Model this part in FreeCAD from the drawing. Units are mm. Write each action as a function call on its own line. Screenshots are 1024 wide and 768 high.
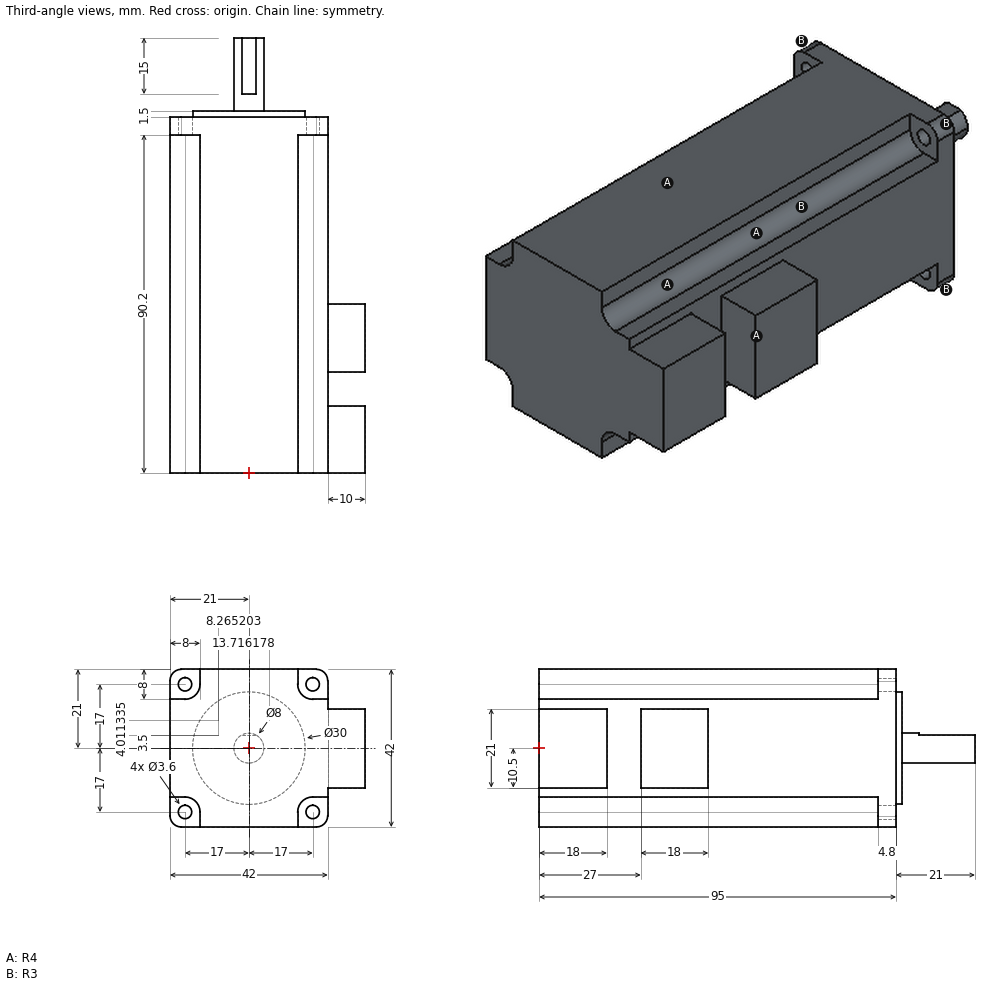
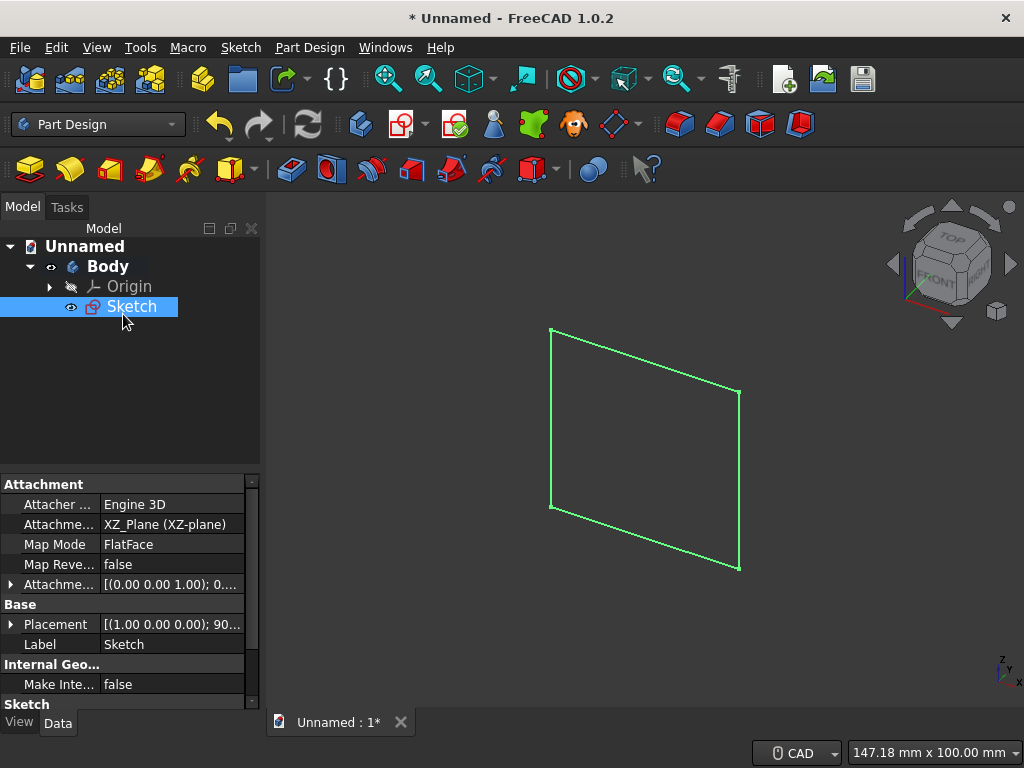
click(30, 170)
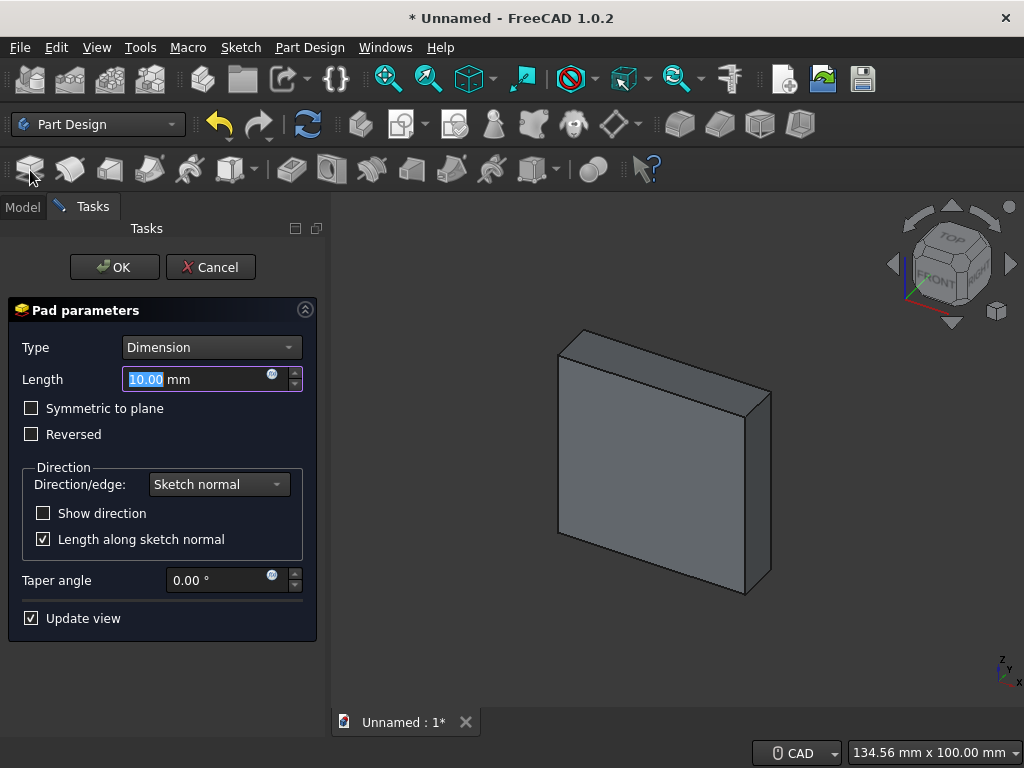
text(95)
key(Tab)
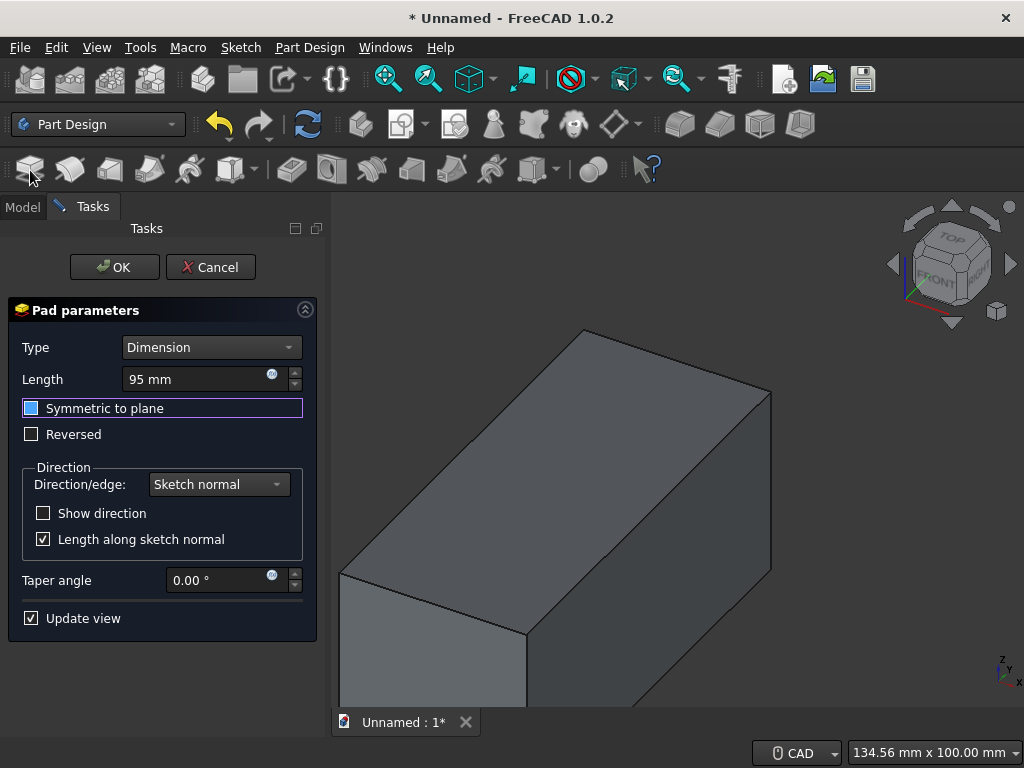
click(30, 434)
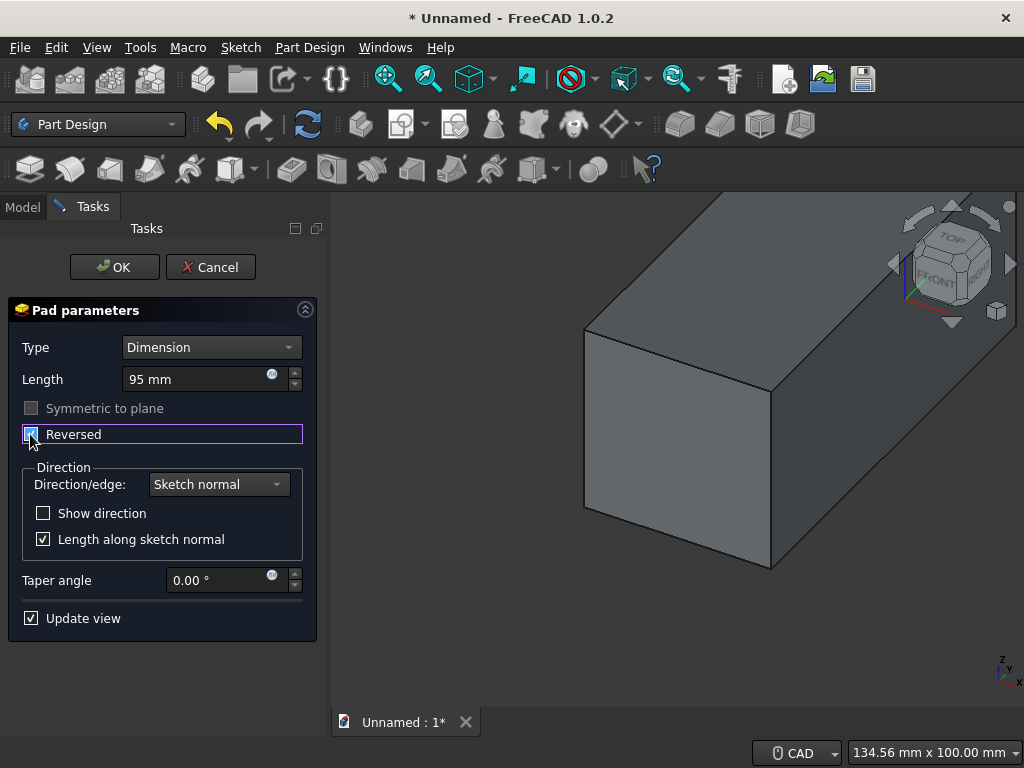
click(115, 267)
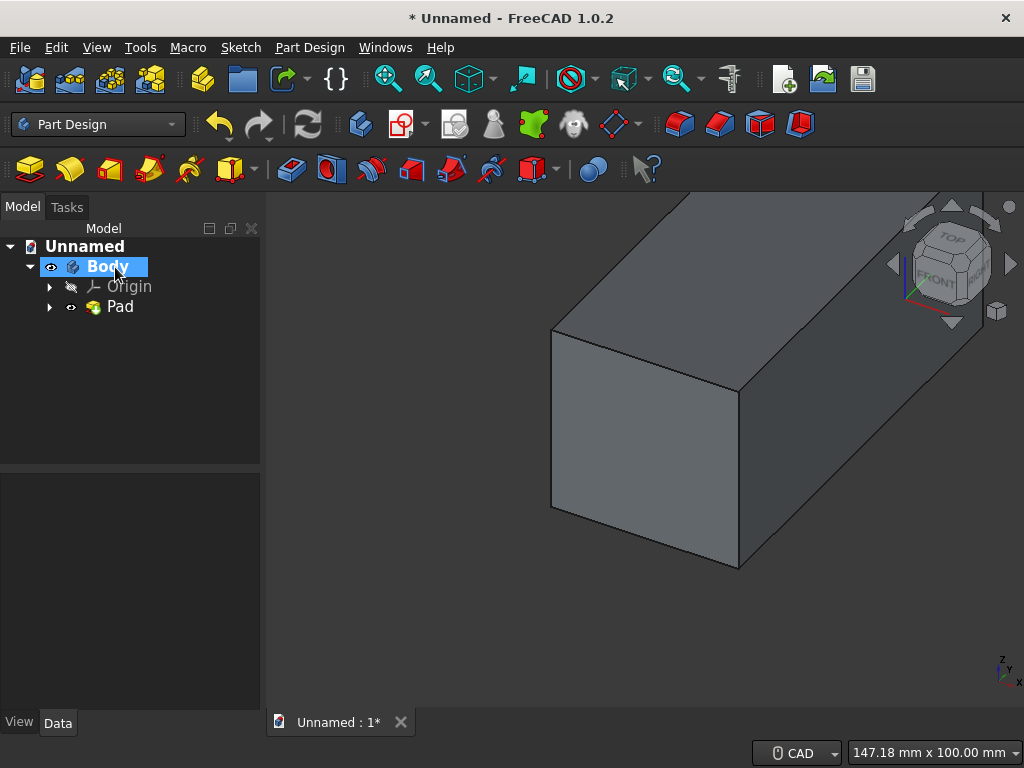
click(390, 80)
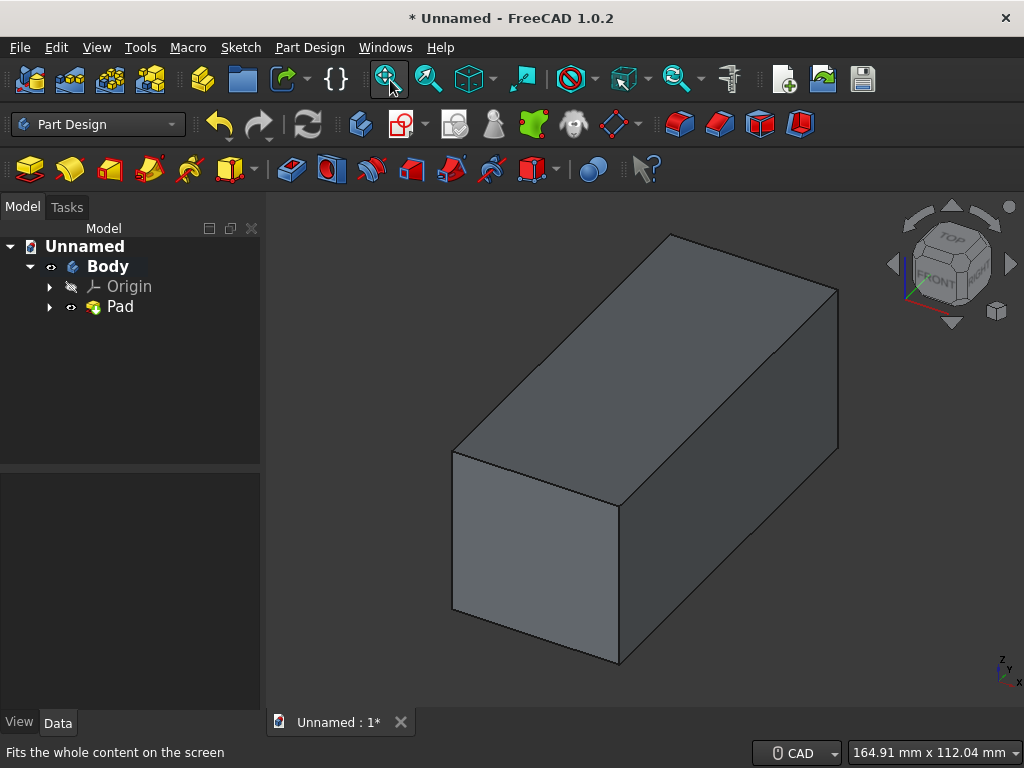
click(536, 557)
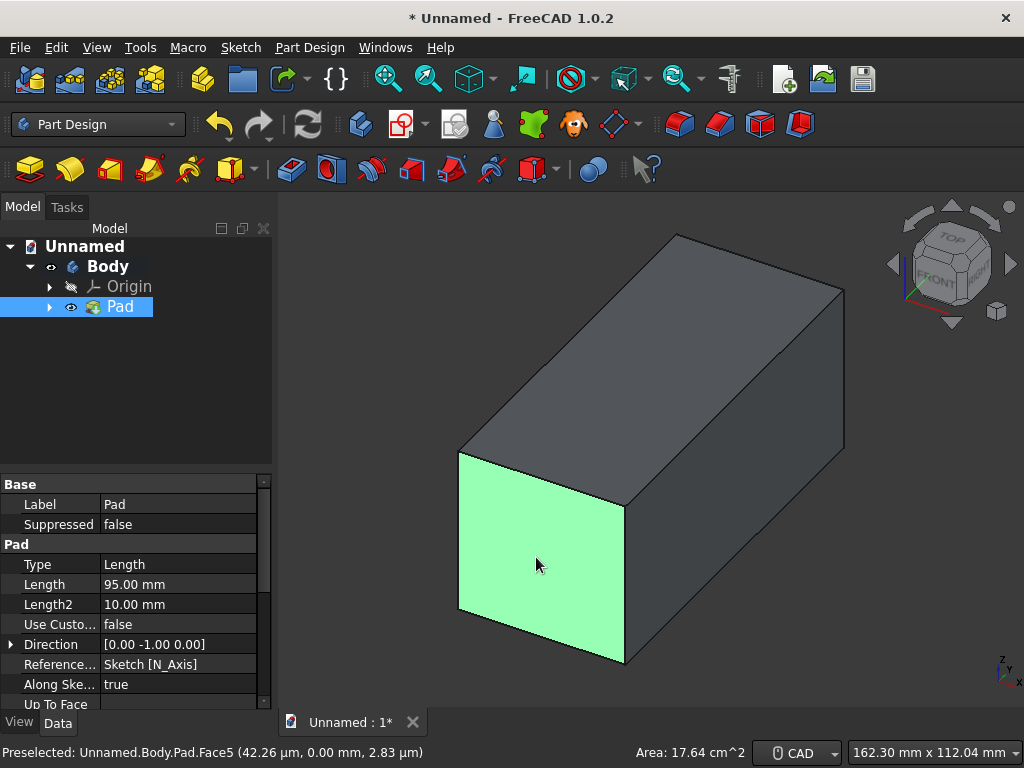
click(402, 124)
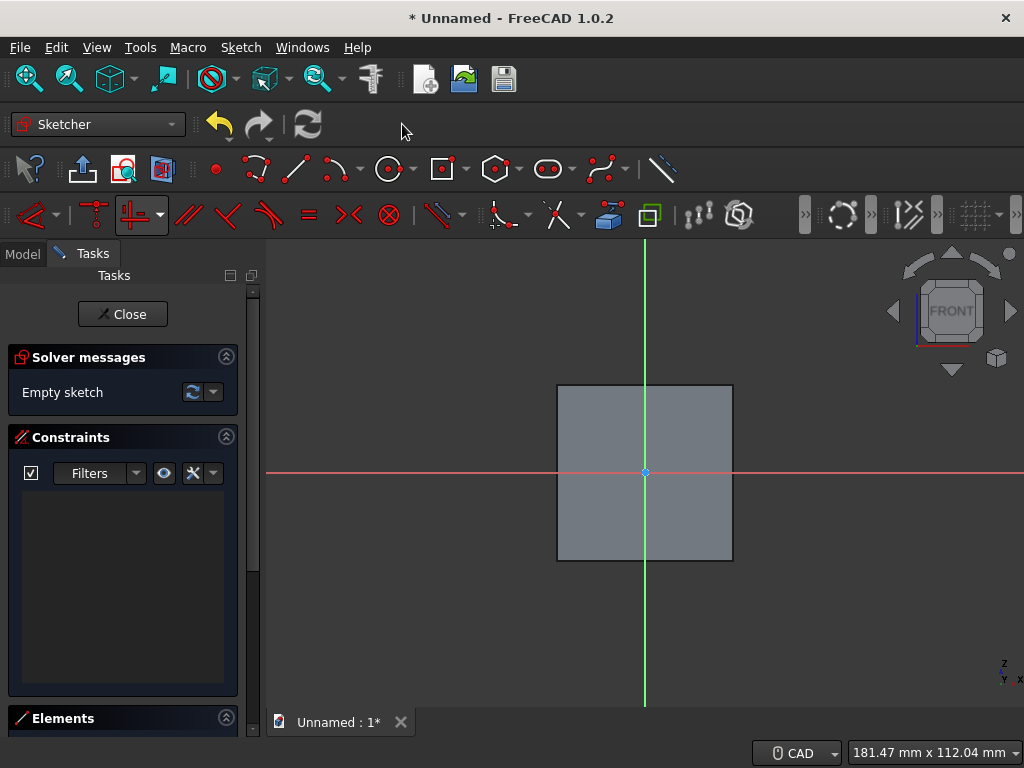
scroll(728, 473, up, 3)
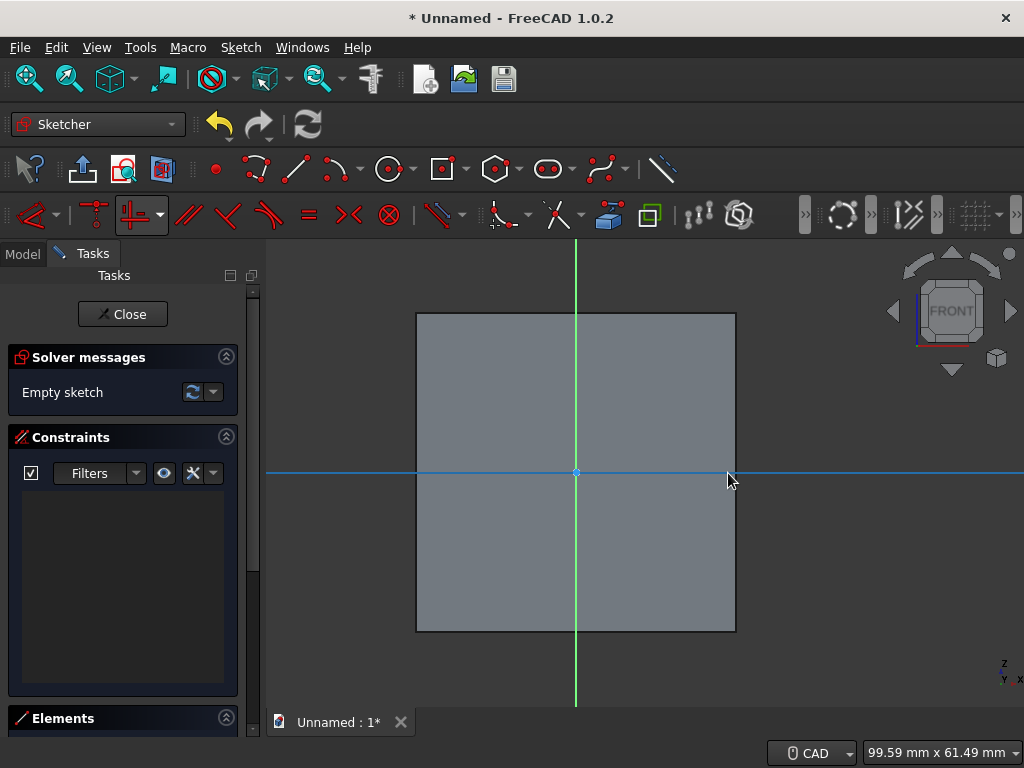
click(468, 170)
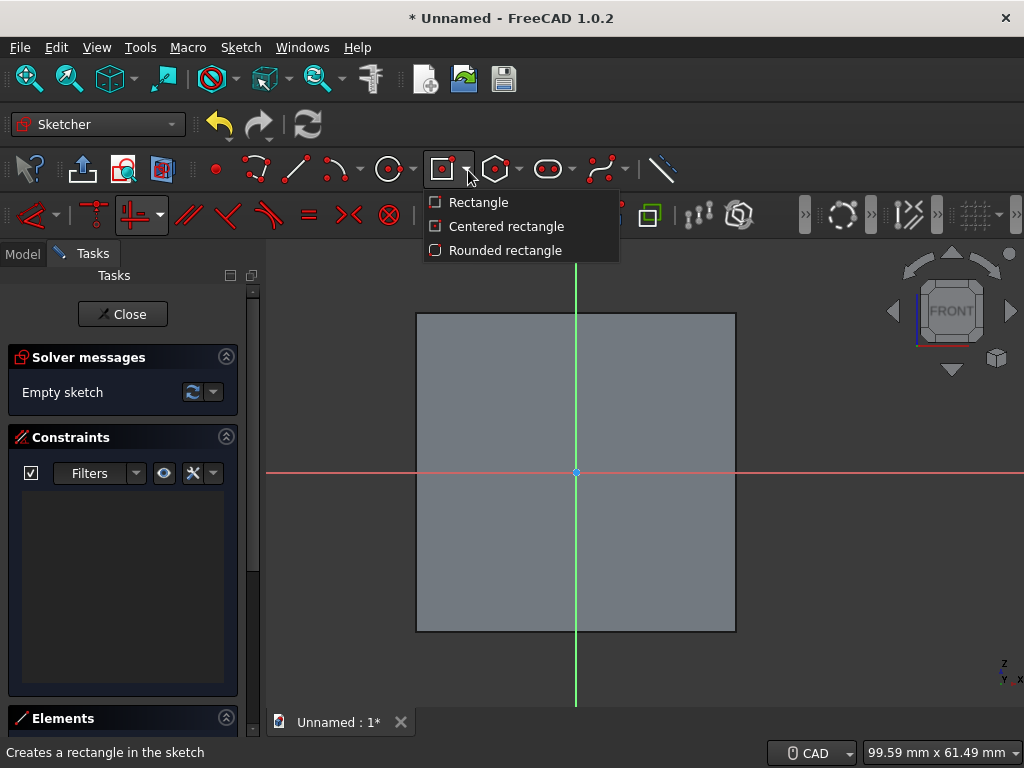
click(522, 202)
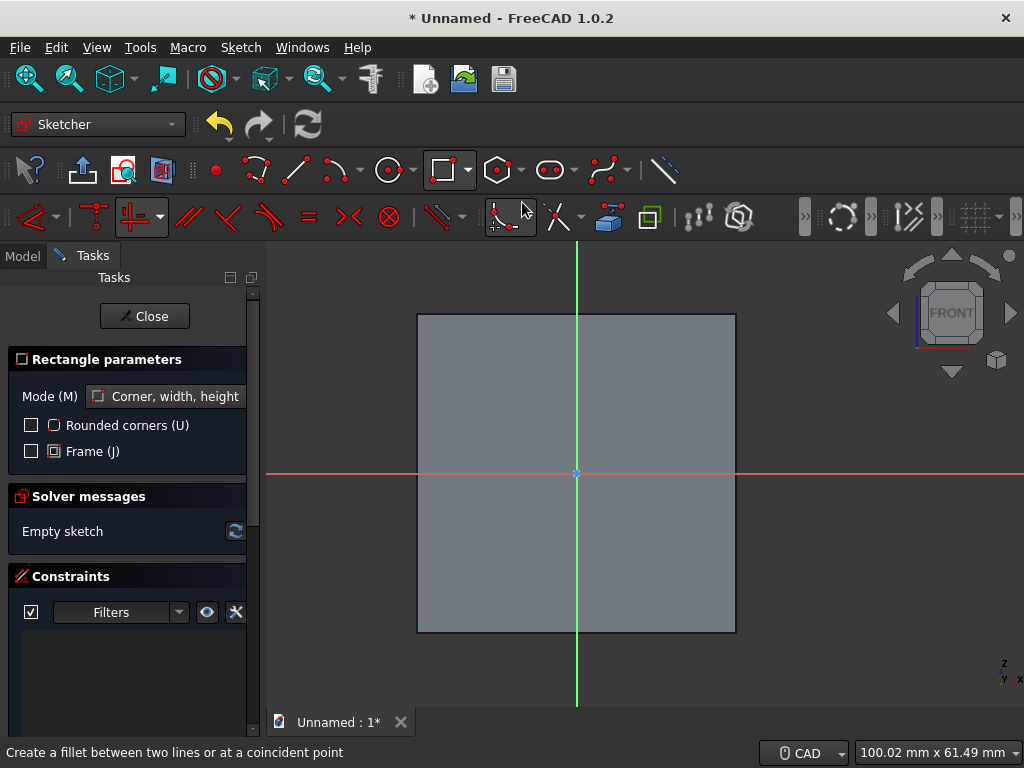
click(417, 314)
click(478, 375)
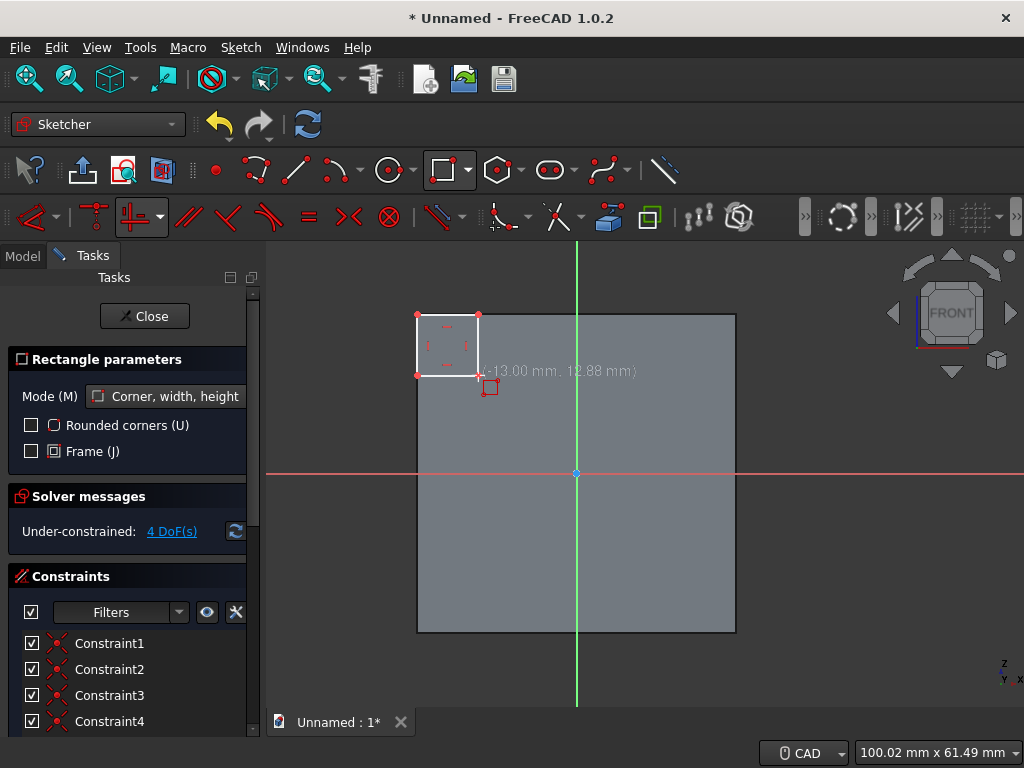
click(675, 314)
click(736, 375)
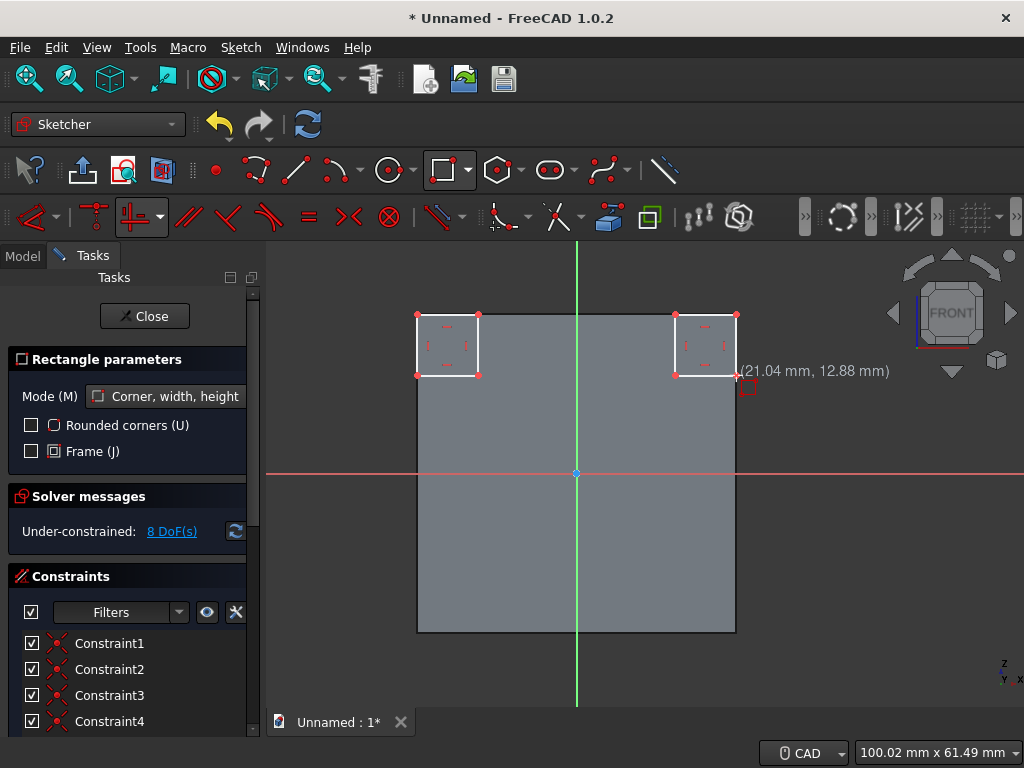
click(417, 572)
click(478, 633)